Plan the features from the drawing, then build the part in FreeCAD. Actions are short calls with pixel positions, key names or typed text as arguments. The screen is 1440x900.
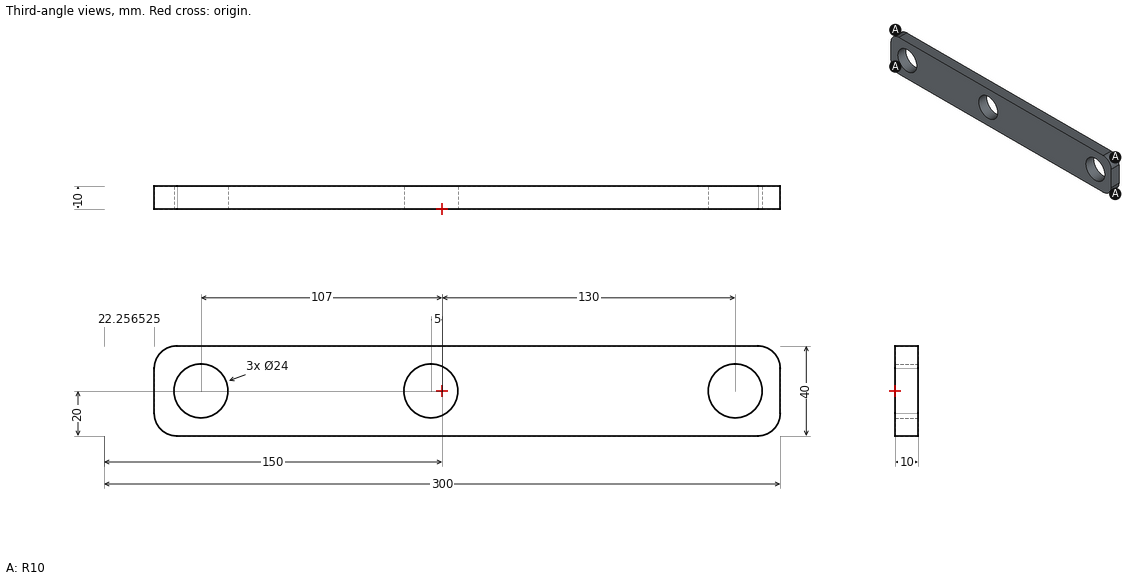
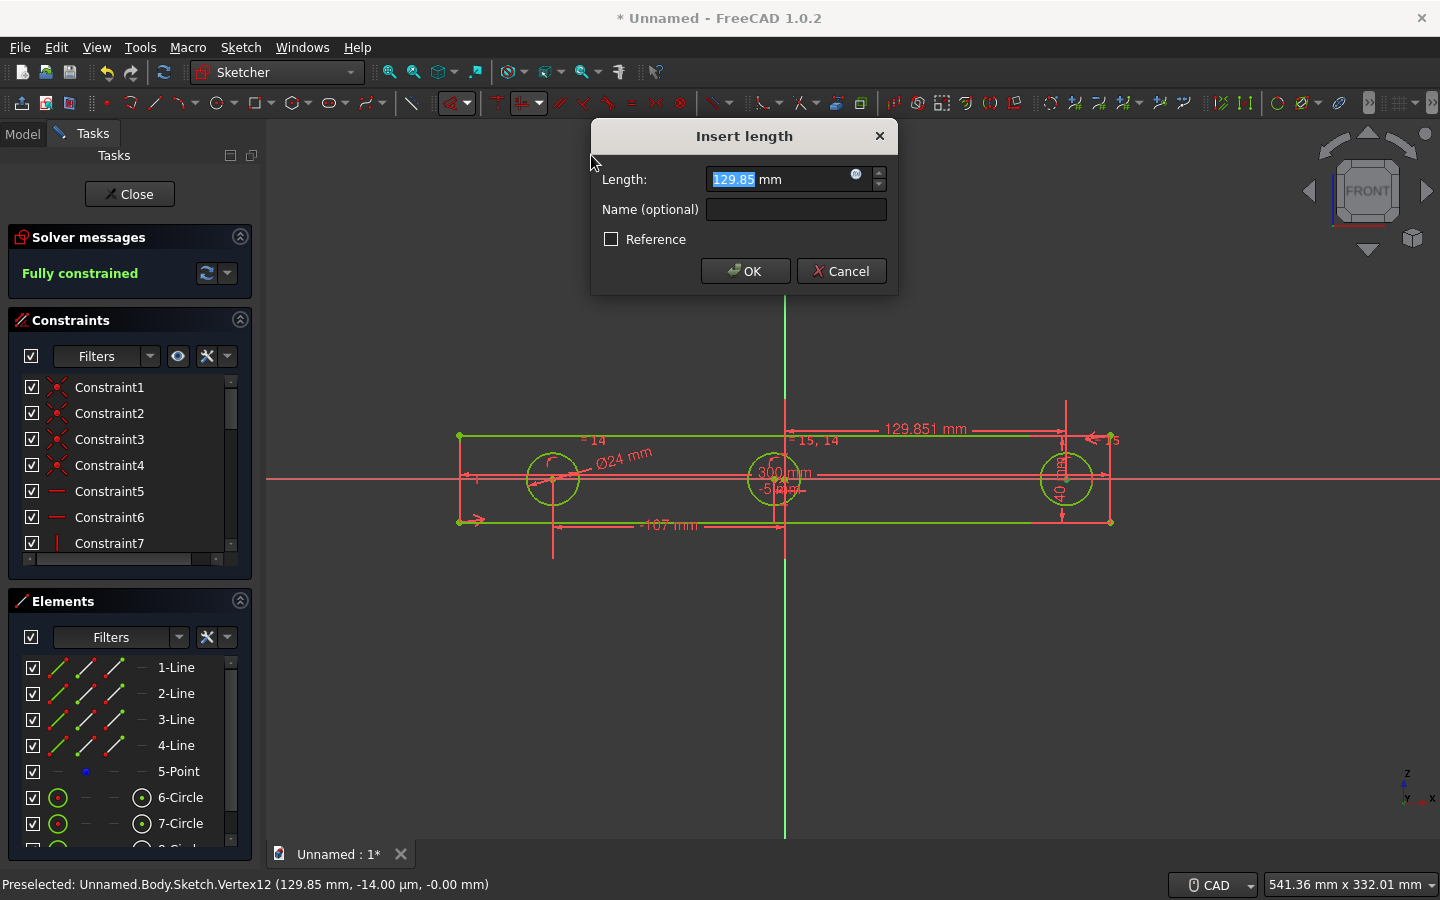
text(130)
key(Return)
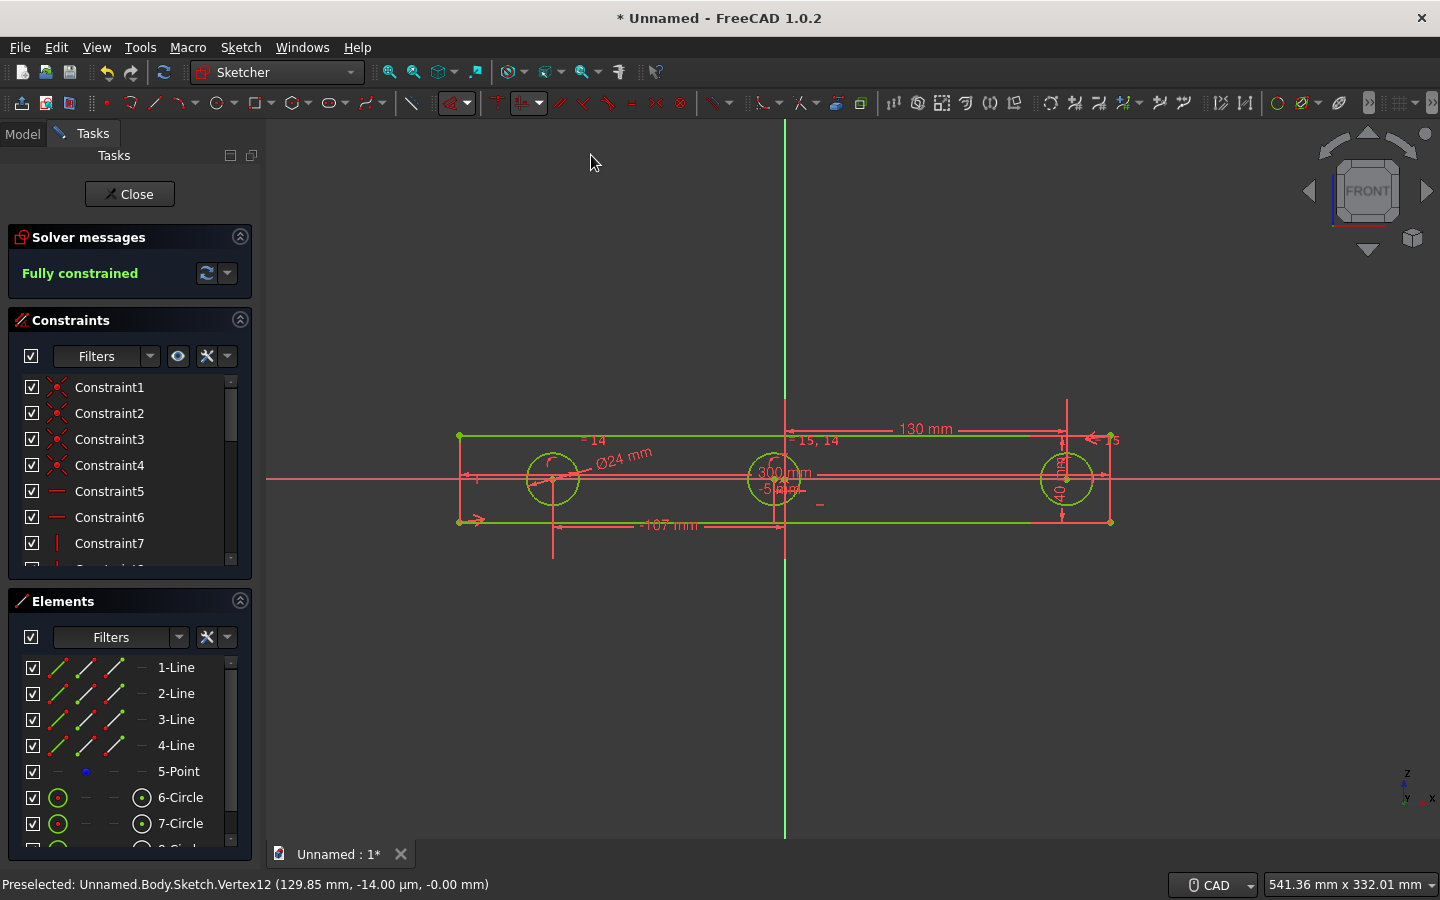
click(130, 194)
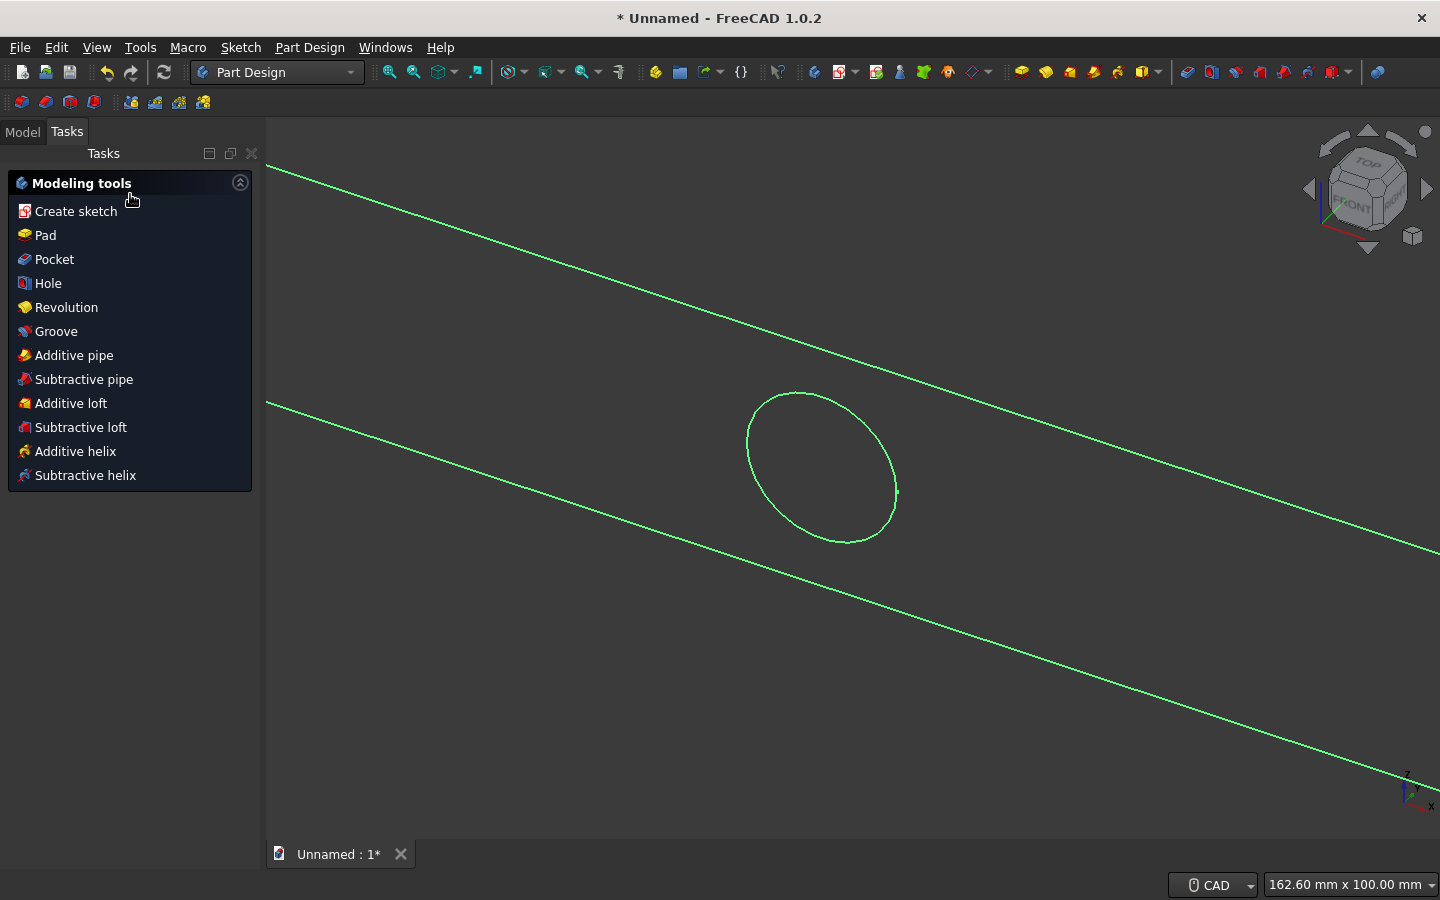
click(1022, 72)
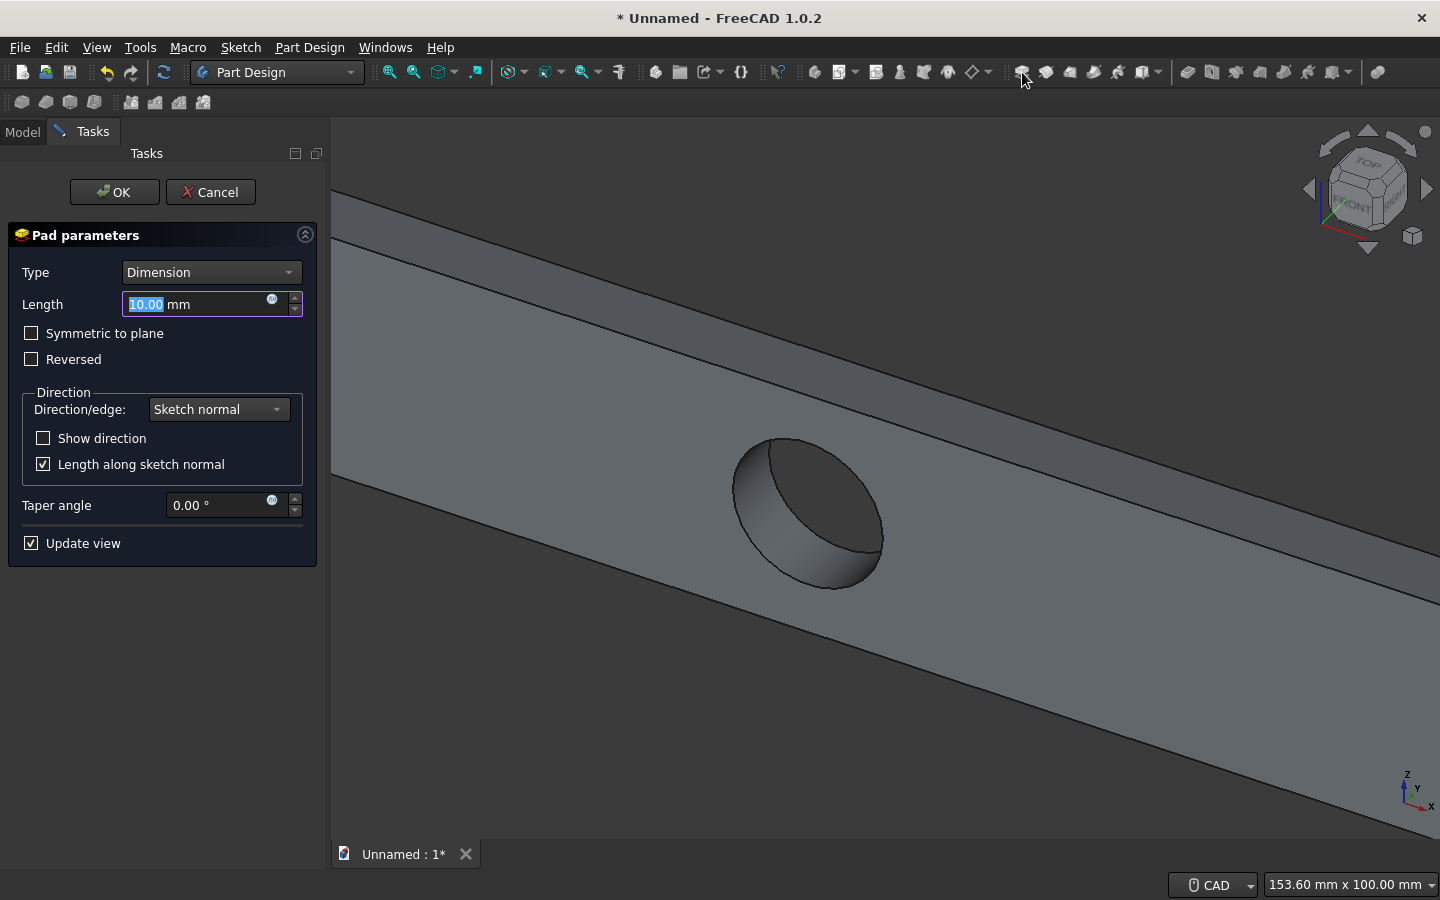
text(10)
key(Tab)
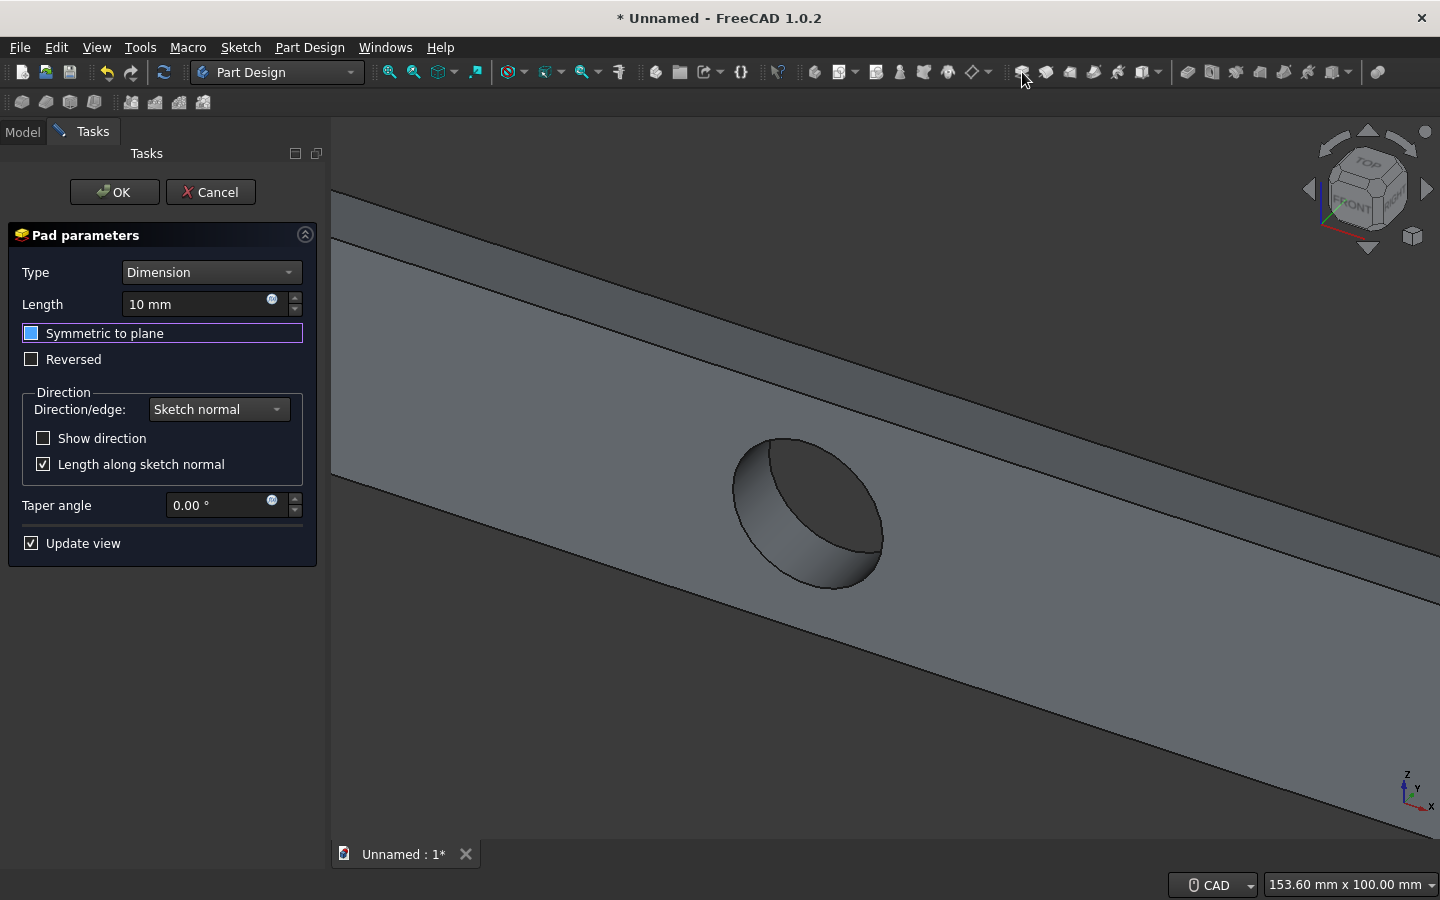
click(30, 359)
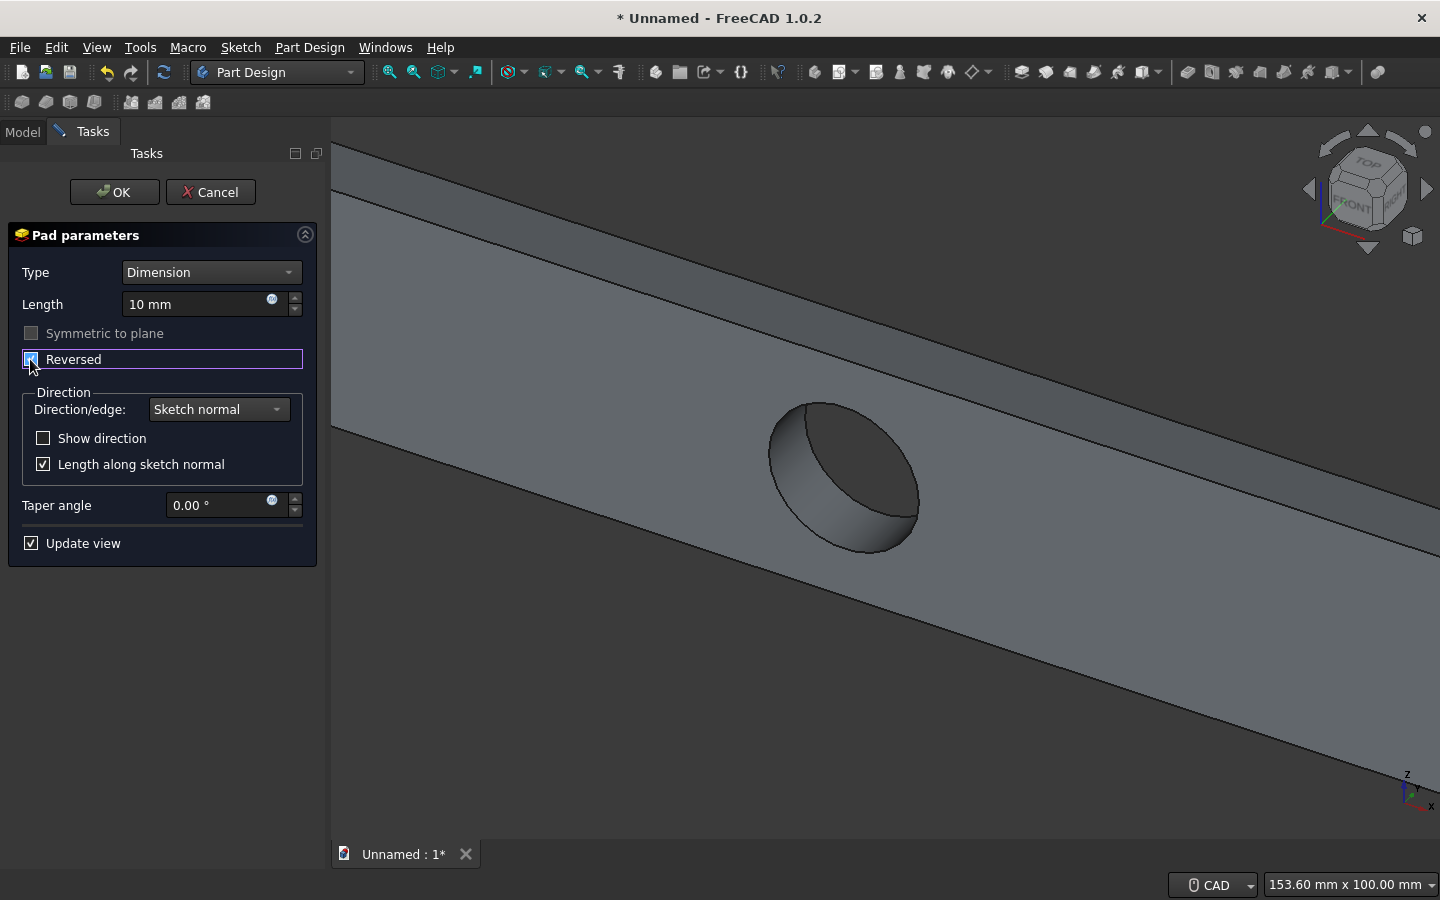
click(115, 192)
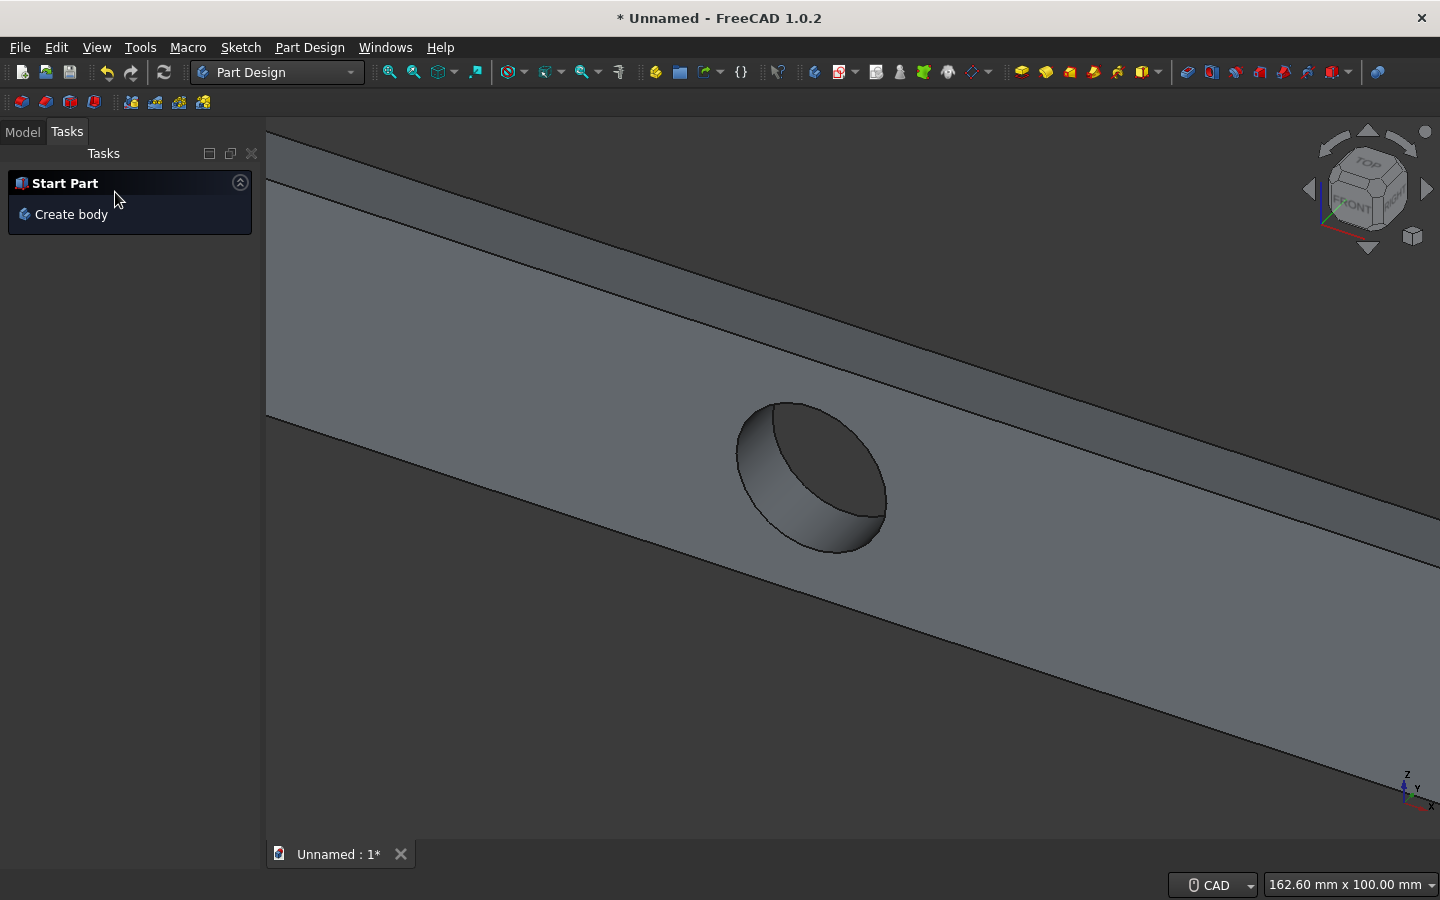
click(390, 72)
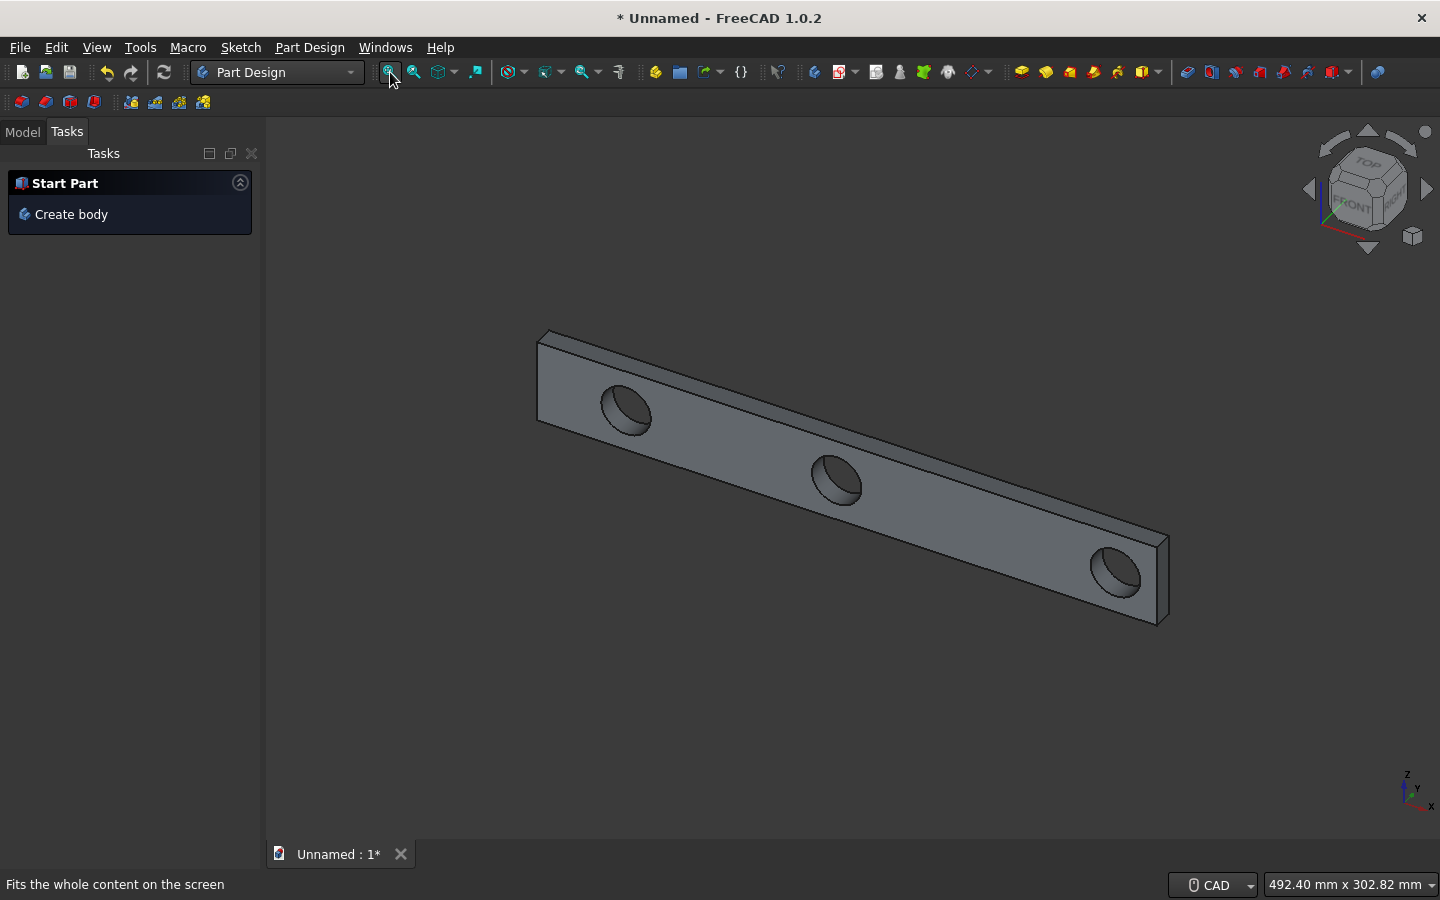
key(4)